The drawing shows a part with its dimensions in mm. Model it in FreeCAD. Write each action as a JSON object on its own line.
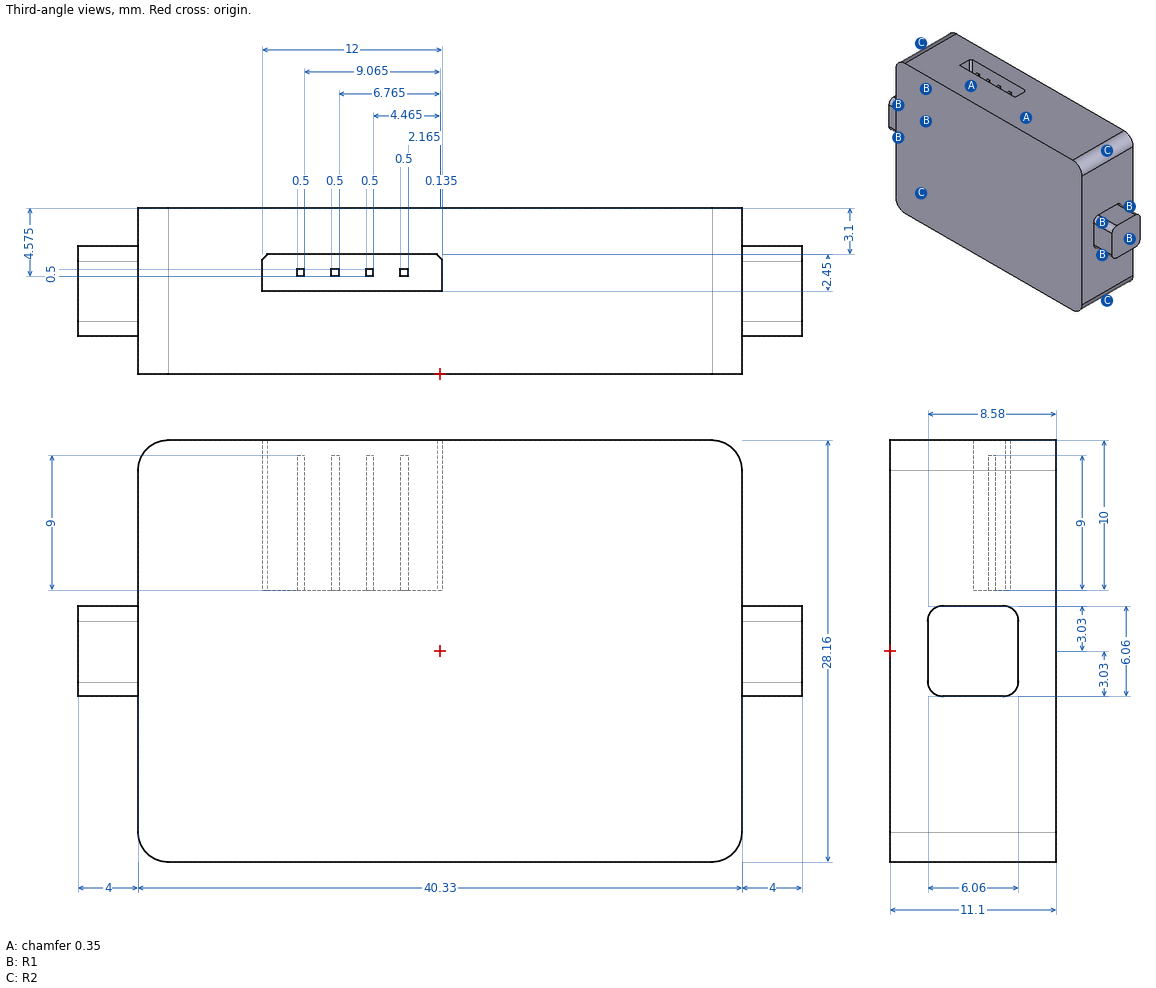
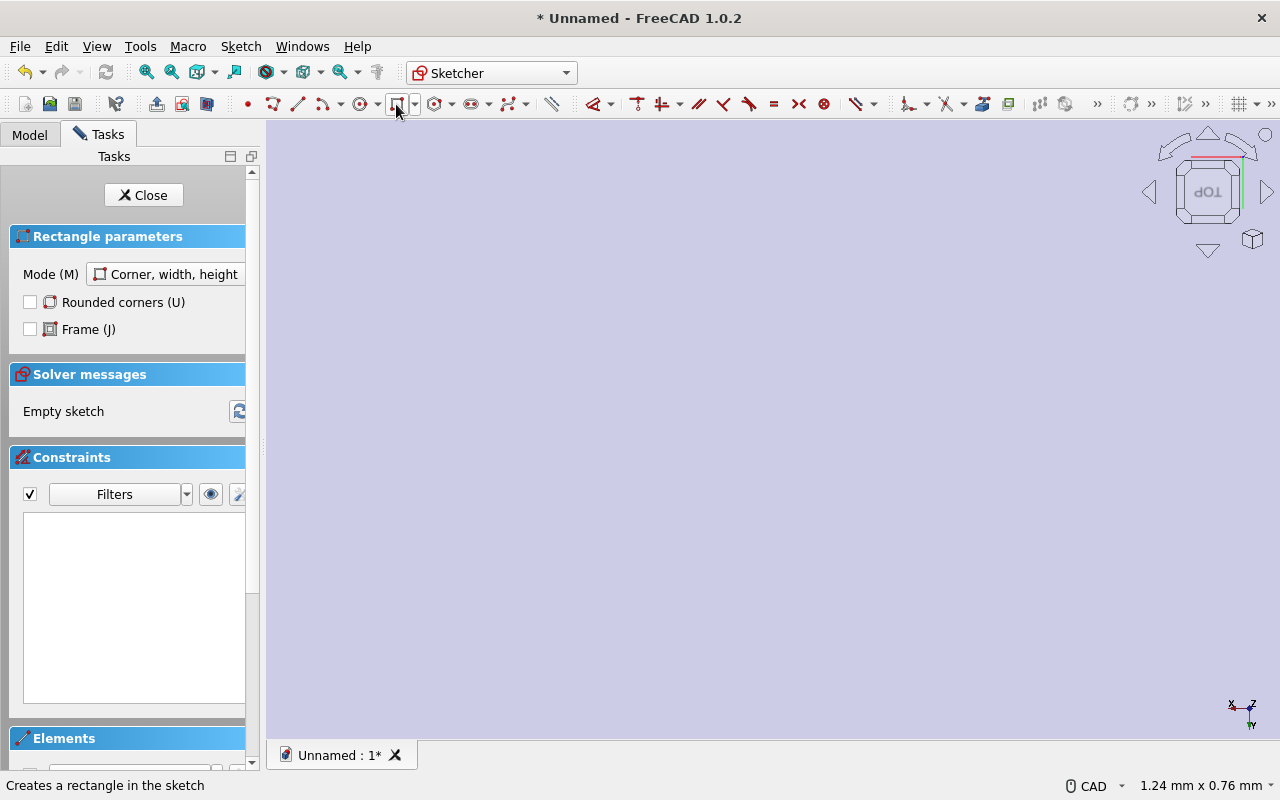
{"action": "left_click", "coordinate": [499, 224]}
{"action": "mouse_move", "coordinate": [909, 633]}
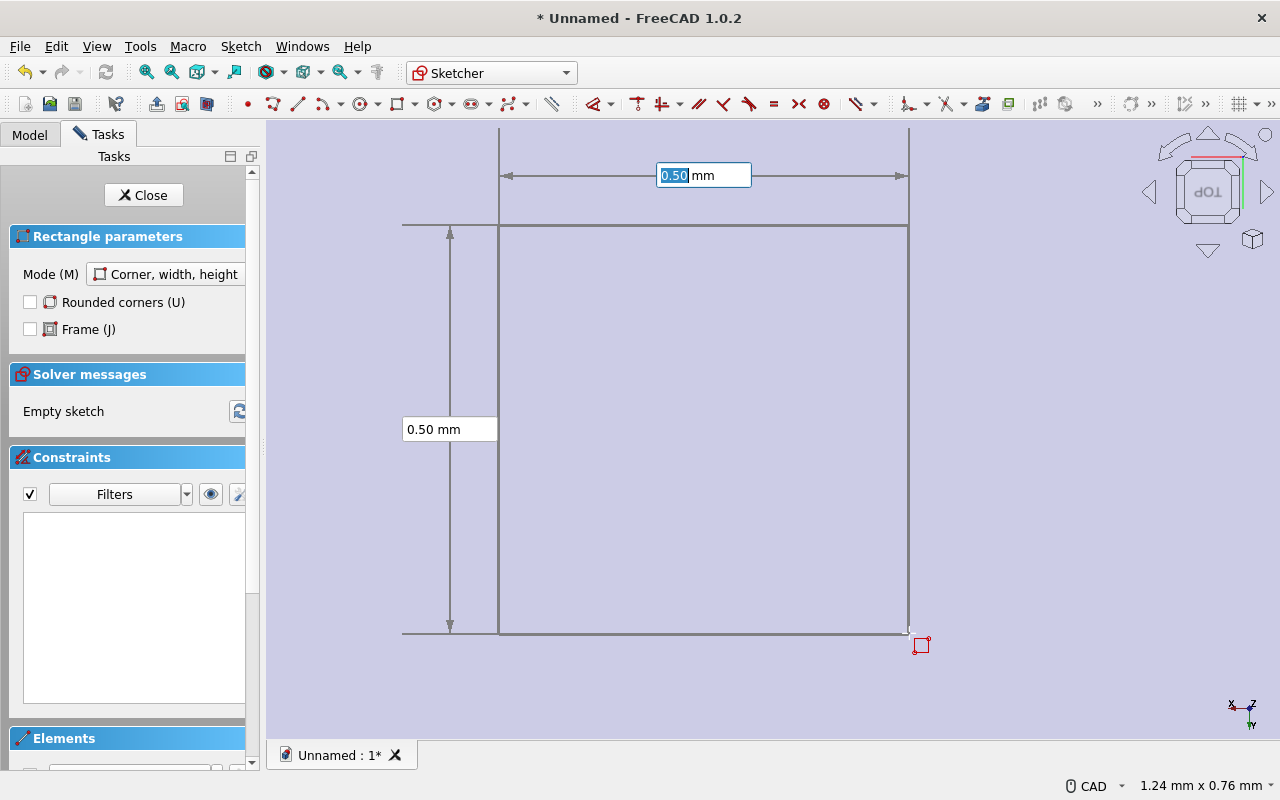
{"action": "type", "text": "0.5"}
{"action": "key", "text": "Tab"}
{"action": "type", "text": "0.5"}
{"action": "key", "text": "Return"}
{"action": "key", "text": "Escape"}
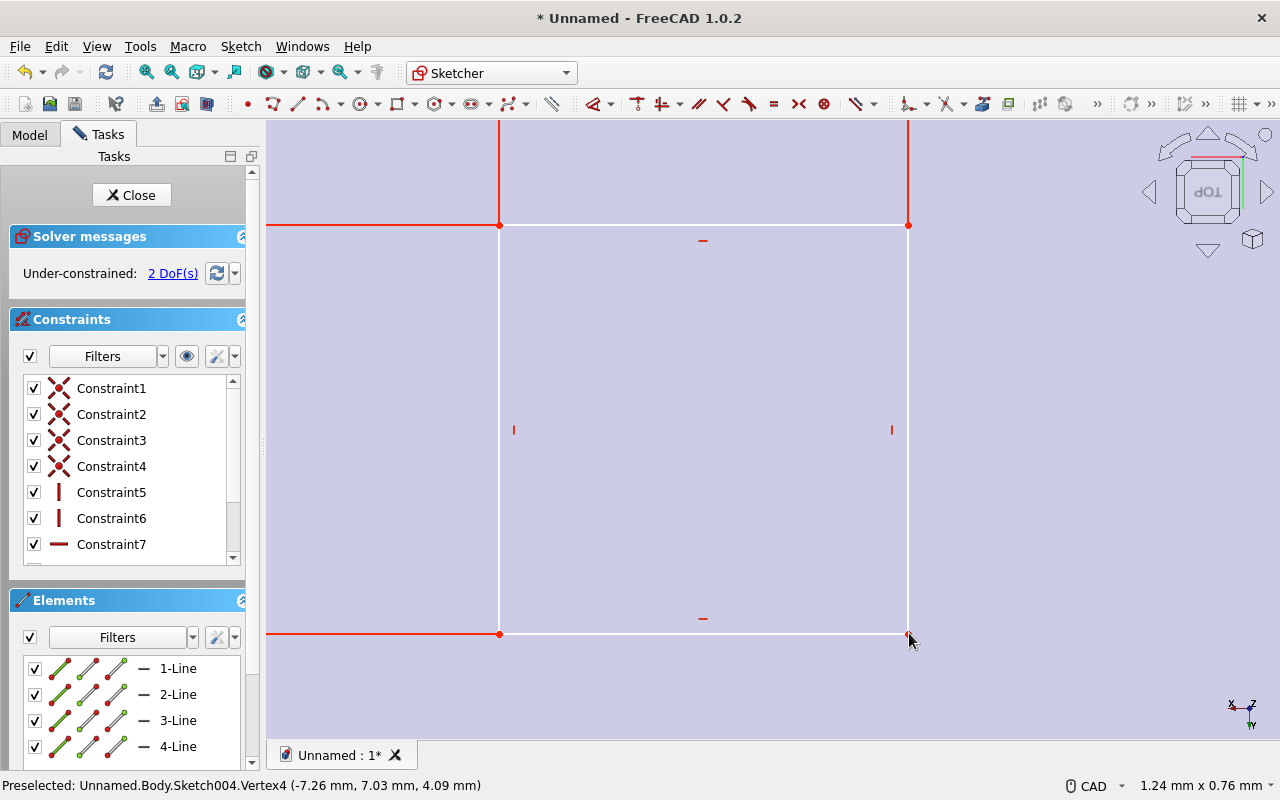
{"action": "left_click", "coordinate": [592, 104]}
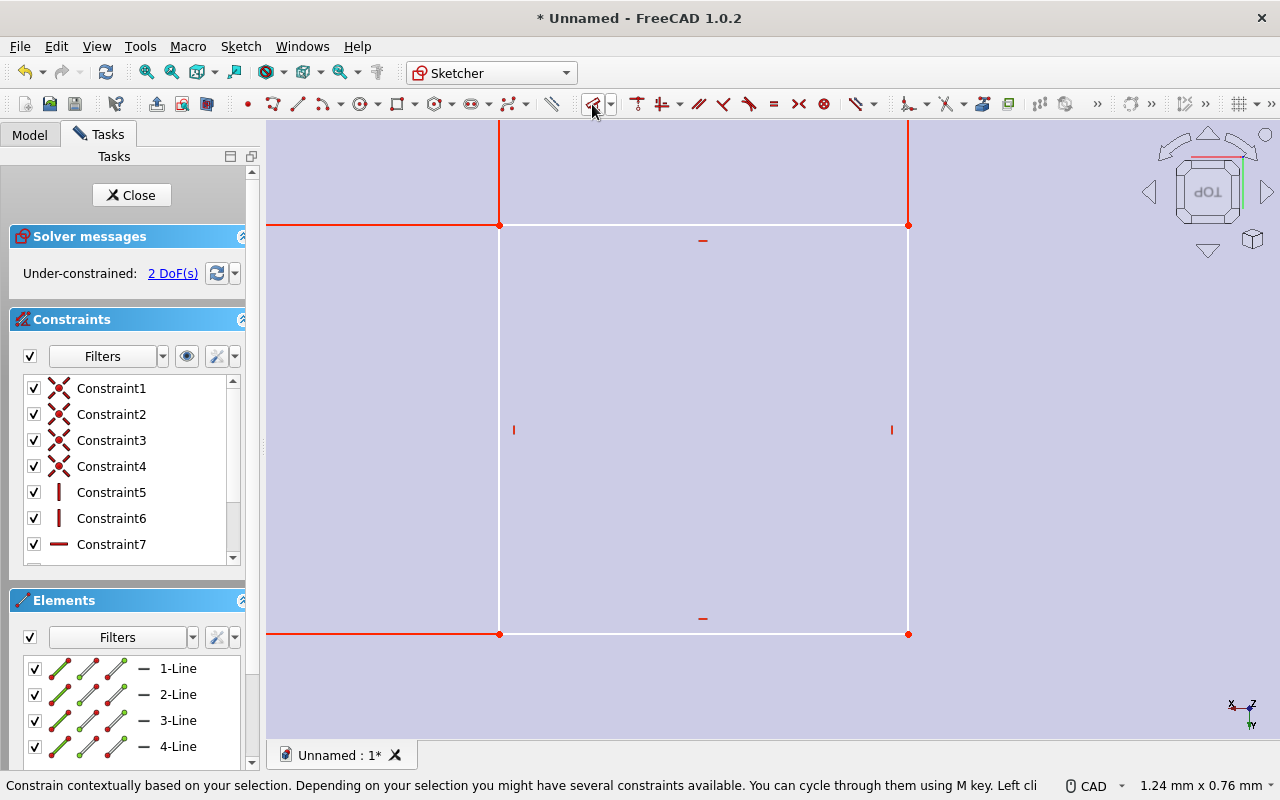
{"action": "left_click", "coordinate": [499, 225]}
{"action": "left_click", "coordinate": [397, 191]}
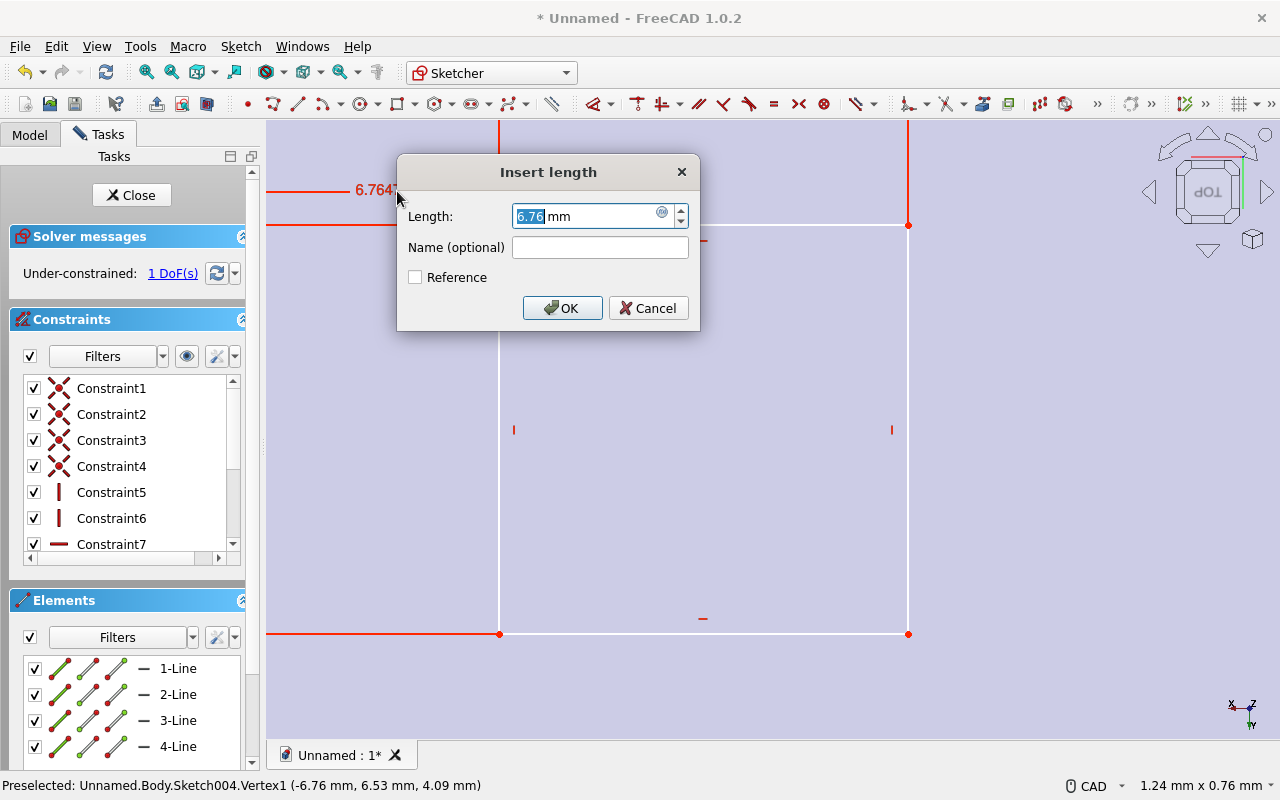
{"action": "type", "text": "6.765"}
{"action": "key", "text": "Return"}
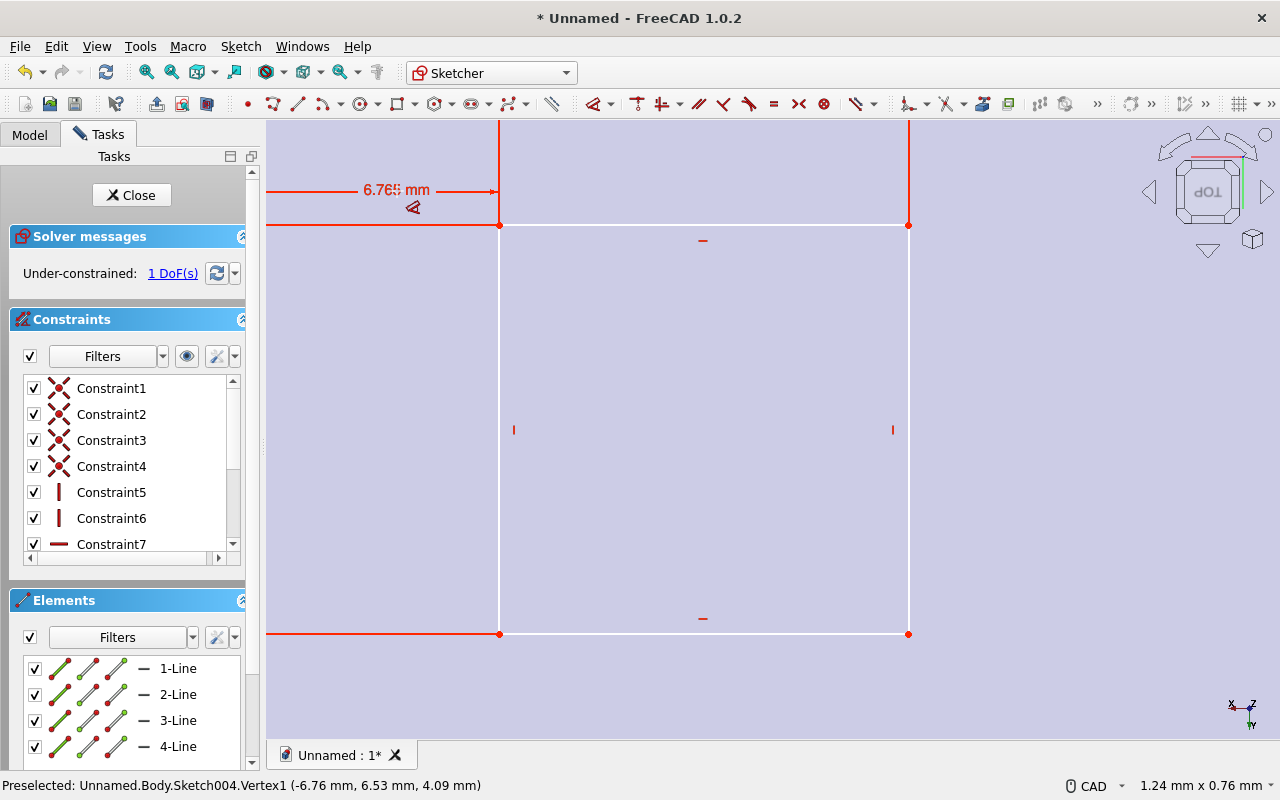
{"action": "left_click", "coordinate": [499, 225]}
{"action": "left_click", "coordinate": [533, 468]}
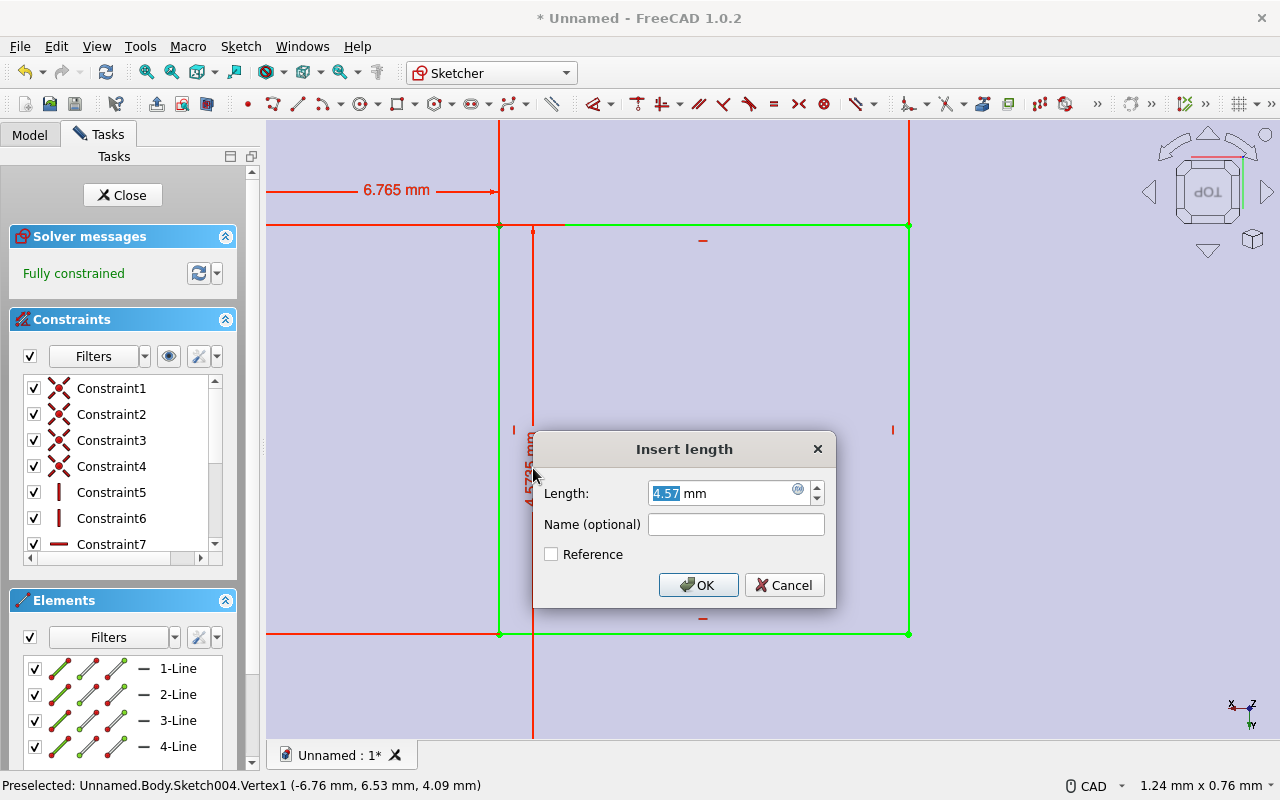
{"action": "type", "text": "4.575"}
{"action": "key", "text": "Return"}
{"action": "key", "text": "Escape"}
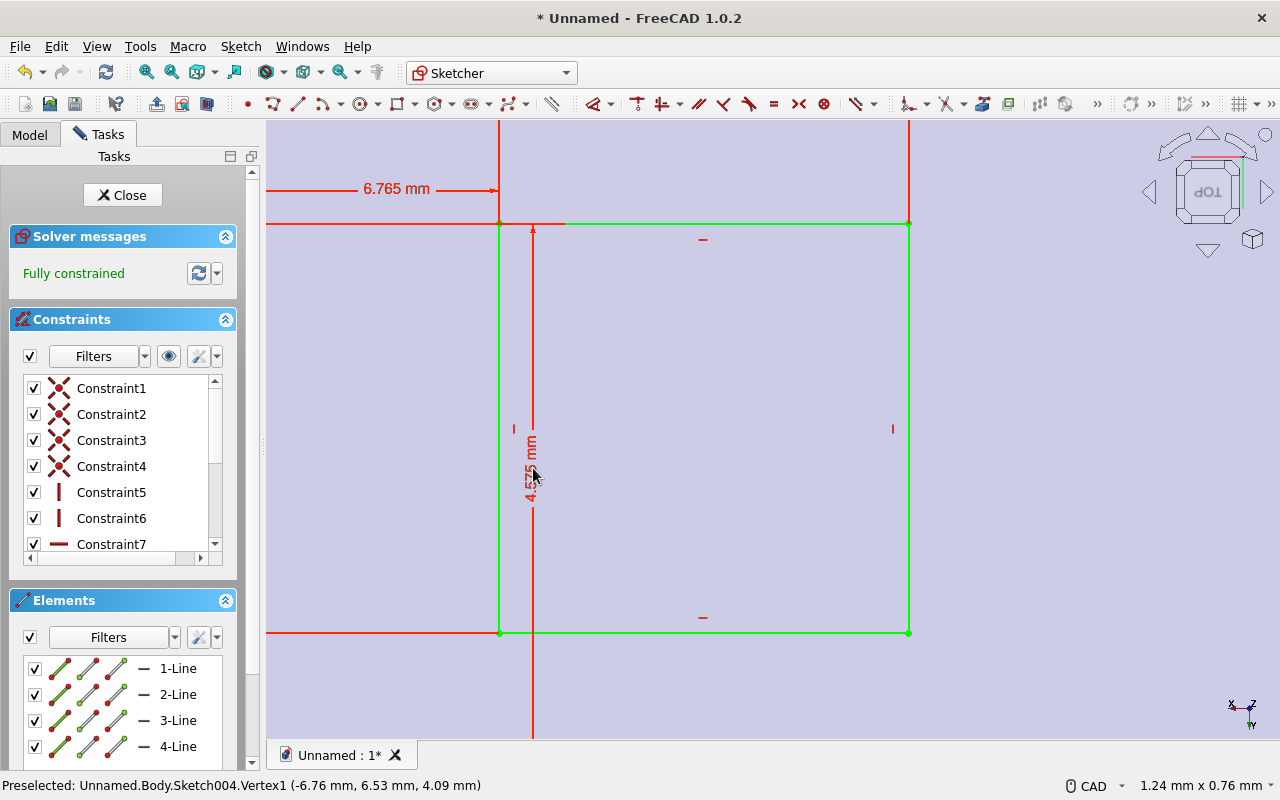
{"action": "left_click", "coordinate": [123, 195]}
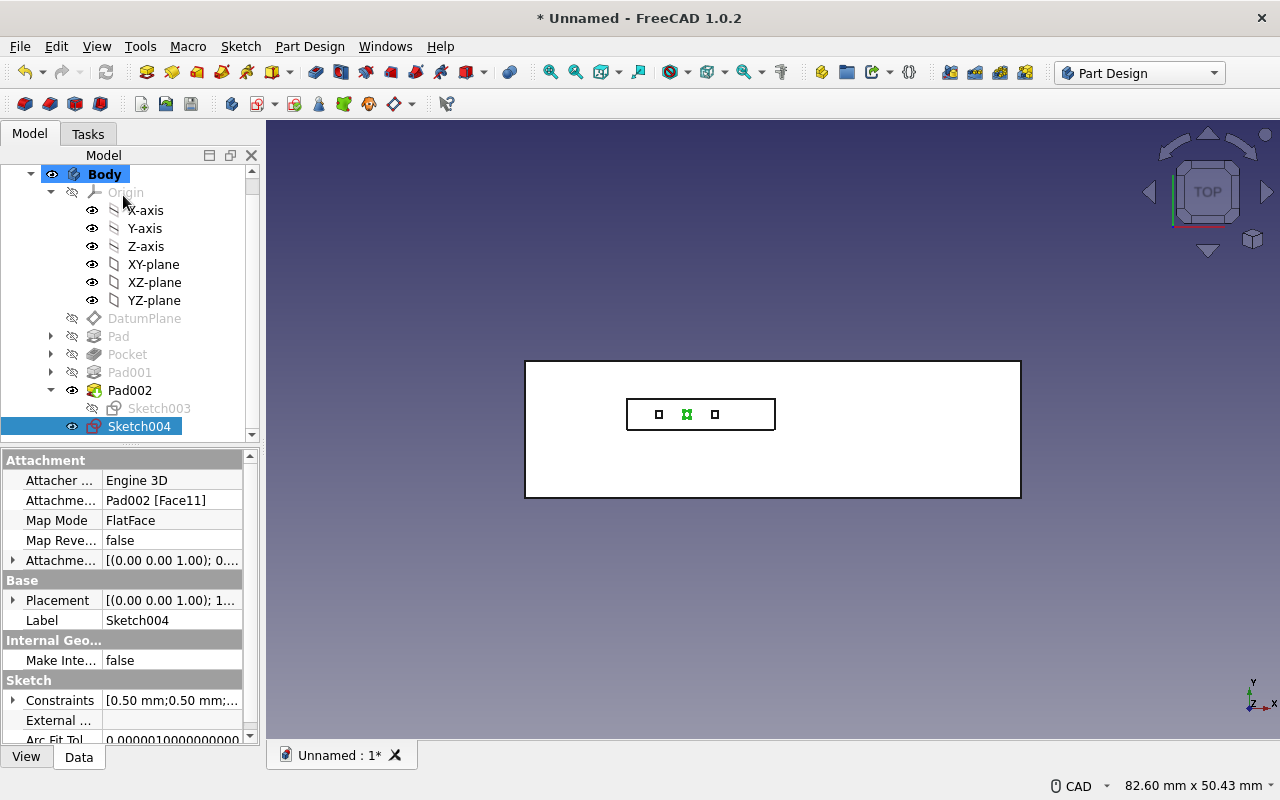
{"action": "left_click", "coordinate": [147, 72]}